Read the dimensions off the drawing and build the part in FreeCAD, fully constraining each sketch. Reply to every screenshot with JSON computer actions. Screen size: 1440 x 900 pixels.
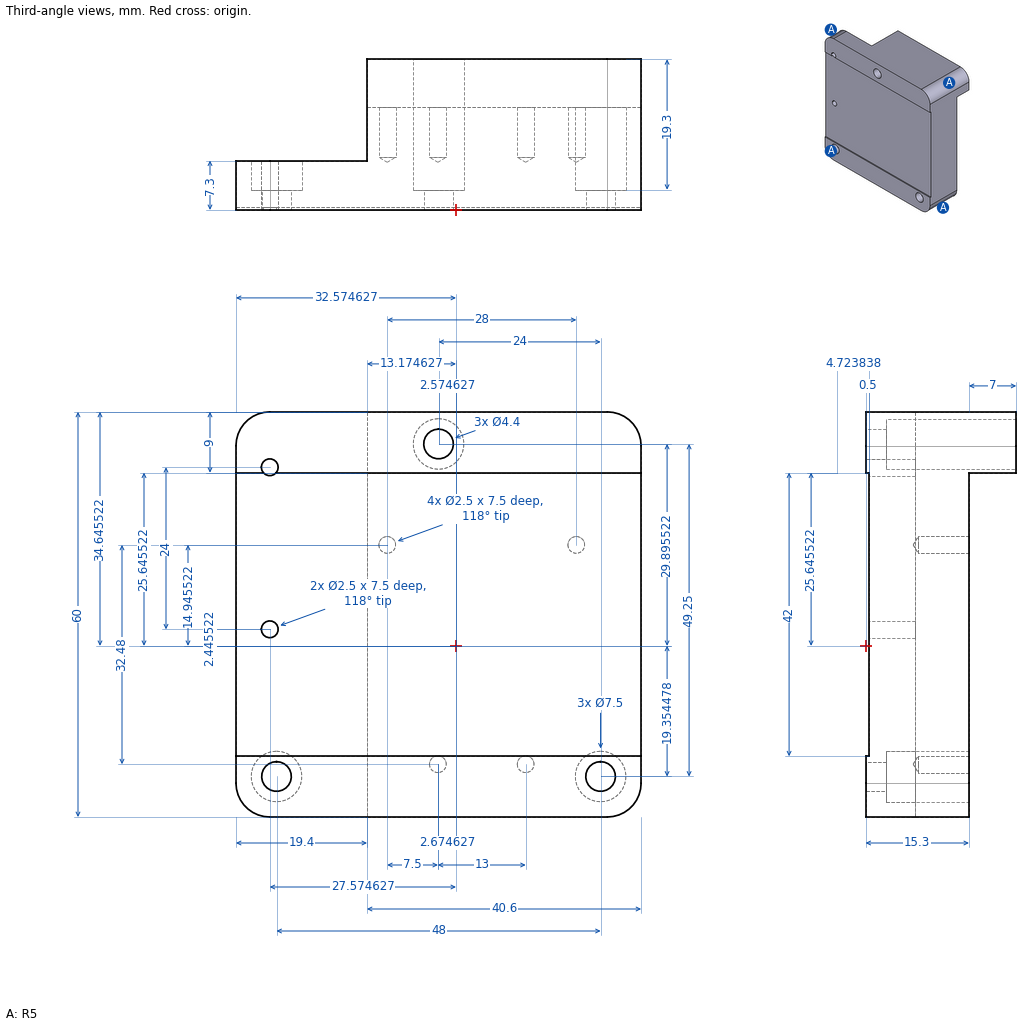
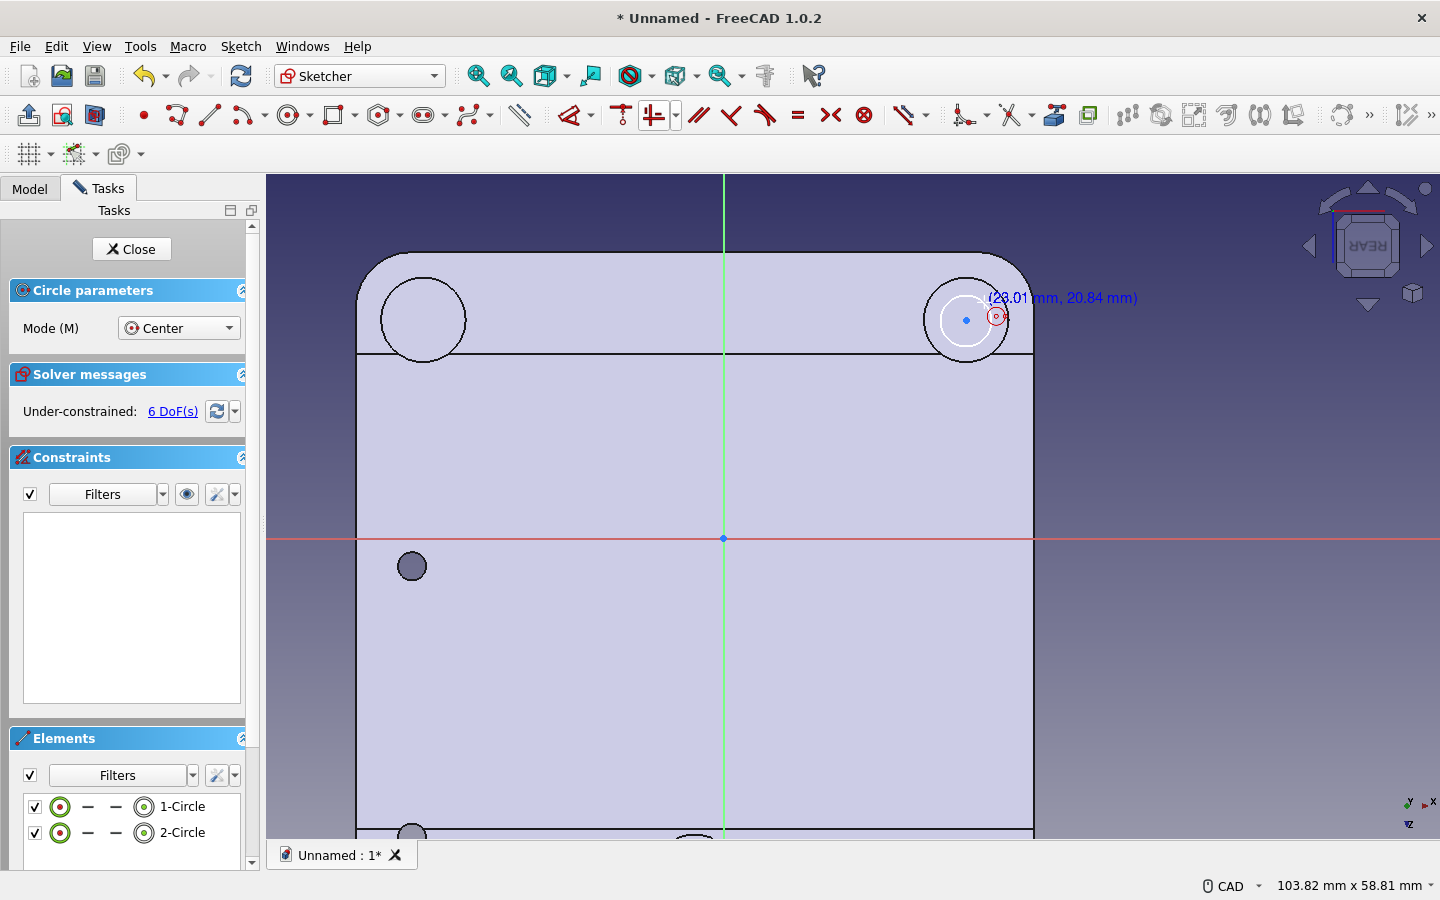
{"action": "left_click", "coordinate": [423, 320]}
{"action": "left_click", "coordinate": [441, 302]}
{"action": "key", "text": "Escape"}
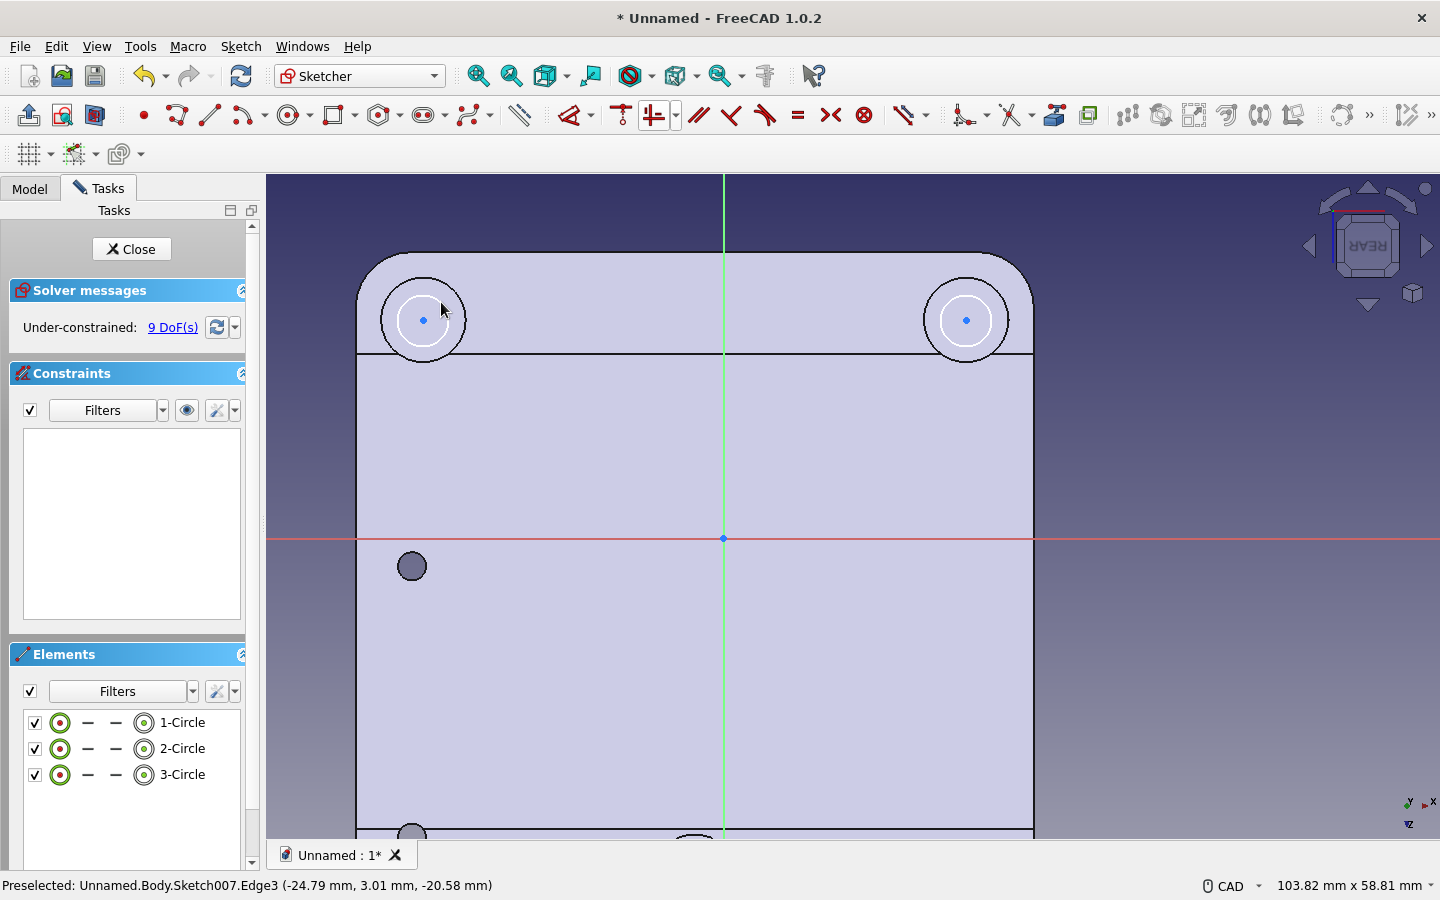
{"action": "scroll", "coordinate": [967, 320], "scroll_direction": "down", "scroll_amount": 2}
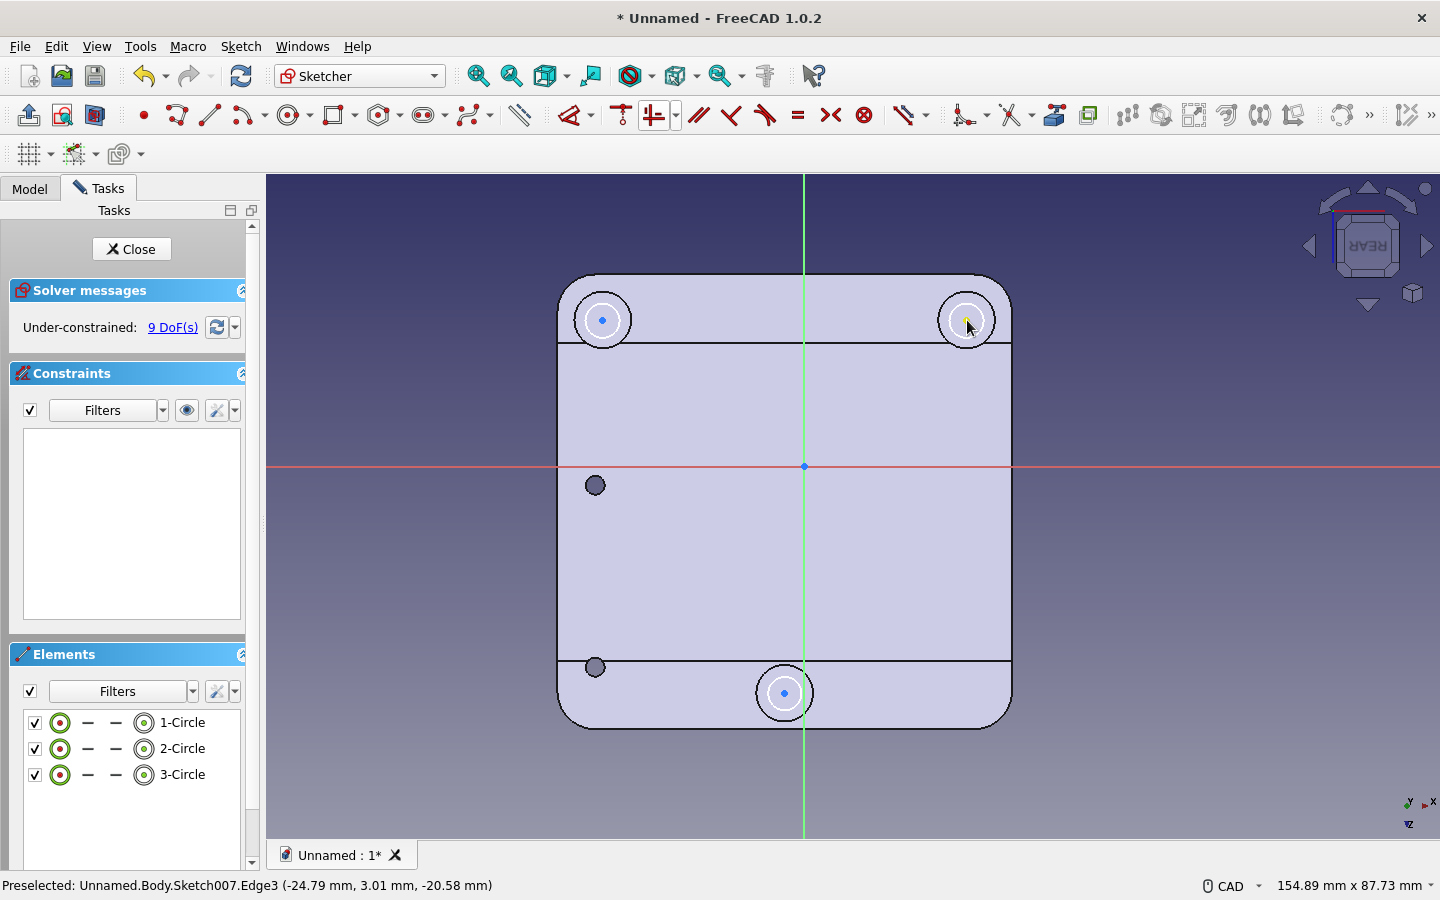
{"action": "scroll", "coordinate": [797, 682], "scroll_direction": "up", "scroll_amount": 3}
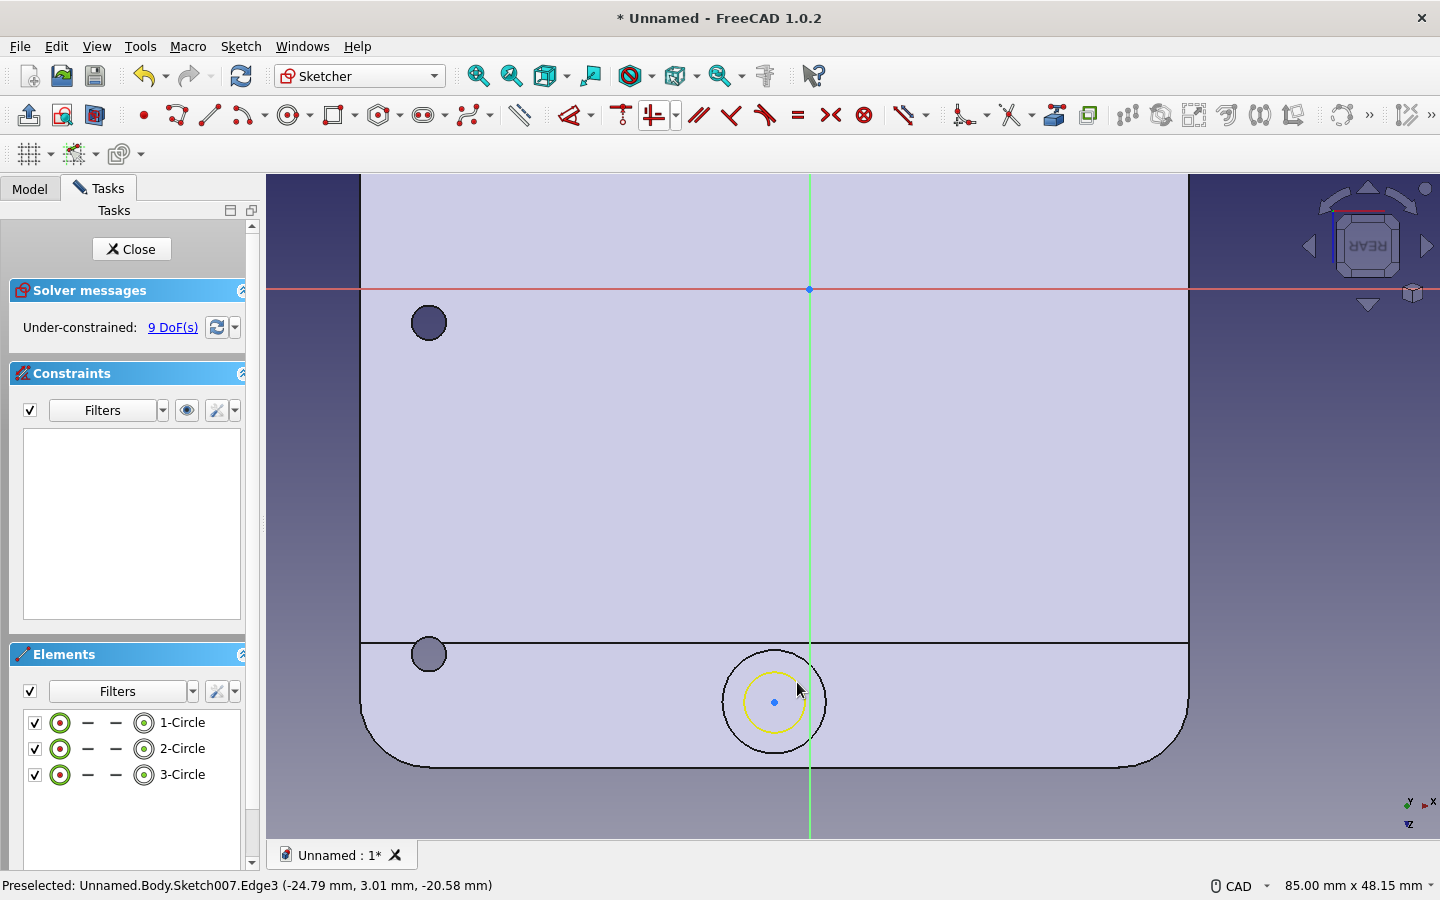
{"action": "left_click", "coordinate": [796, 681]}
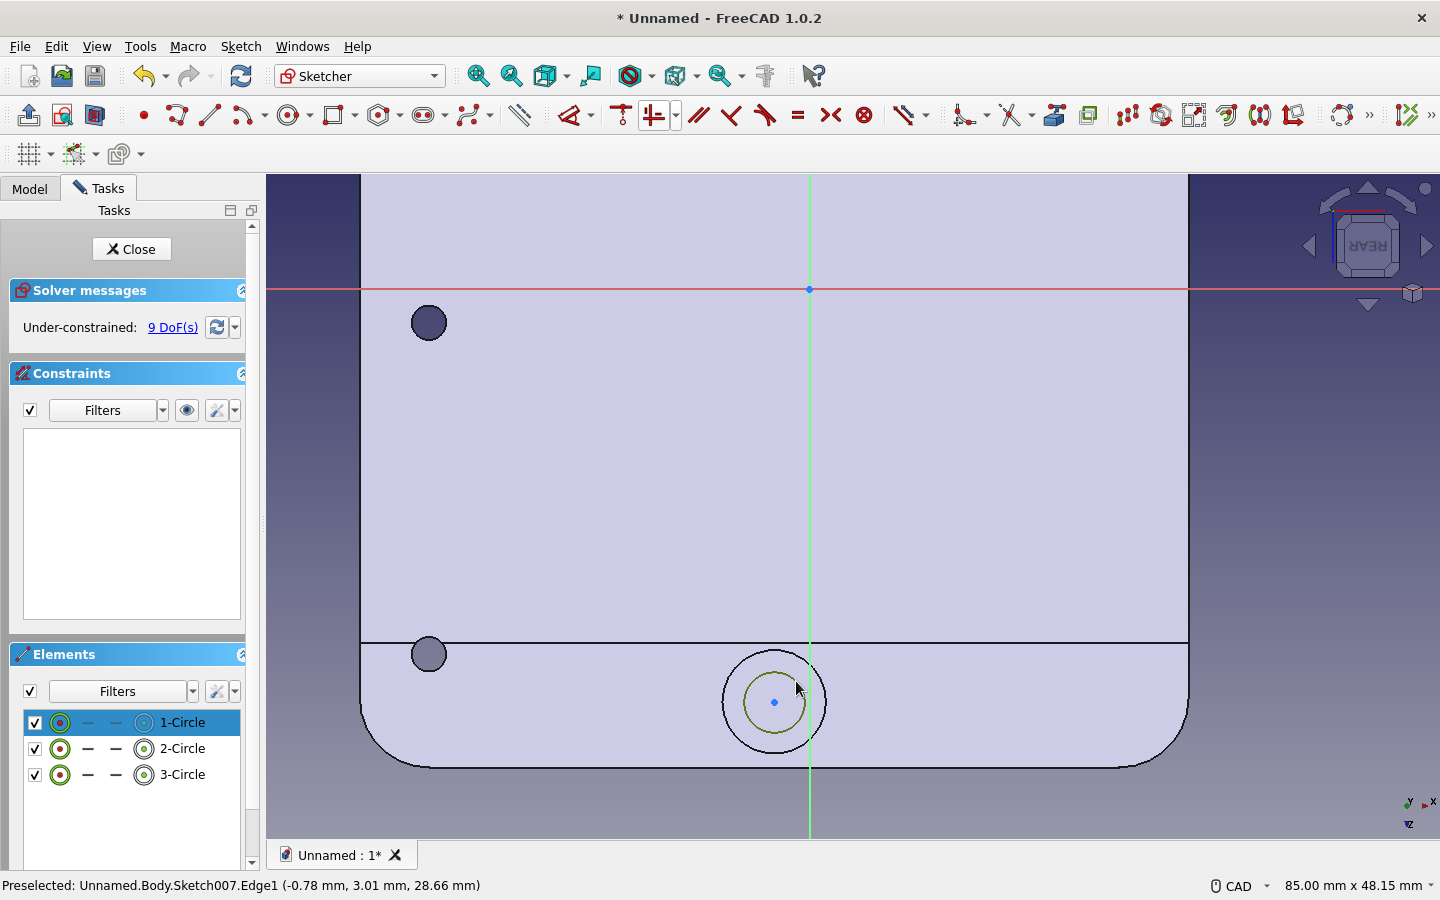
{"action": "scroll", "coordinate": [797, 683], "scroll_direction": "down", "scroll_amount": 3}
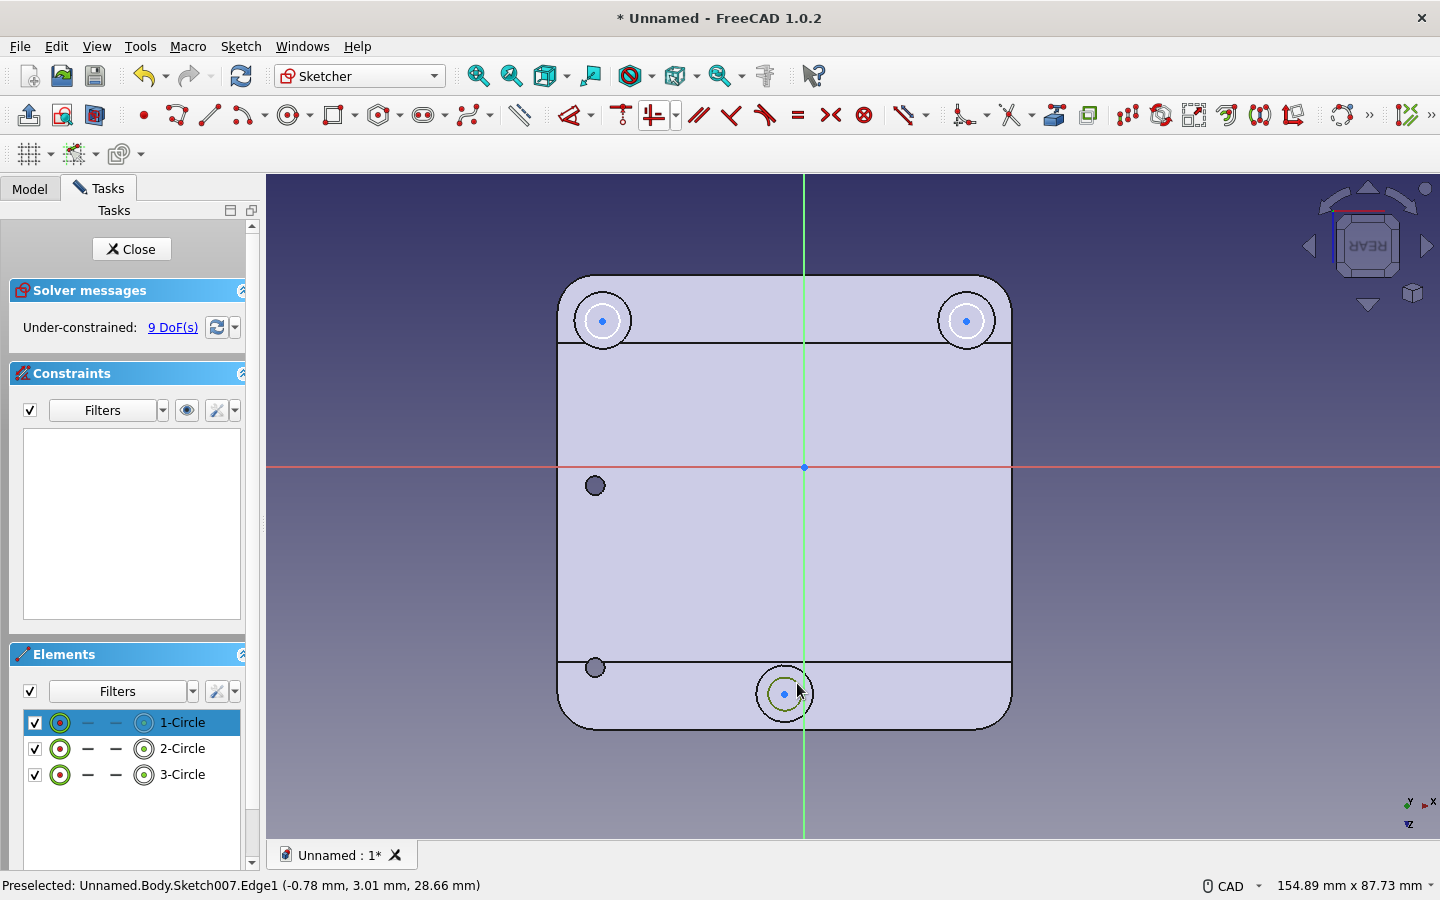
{"action": "left_click", "coordinate": [979, 309]}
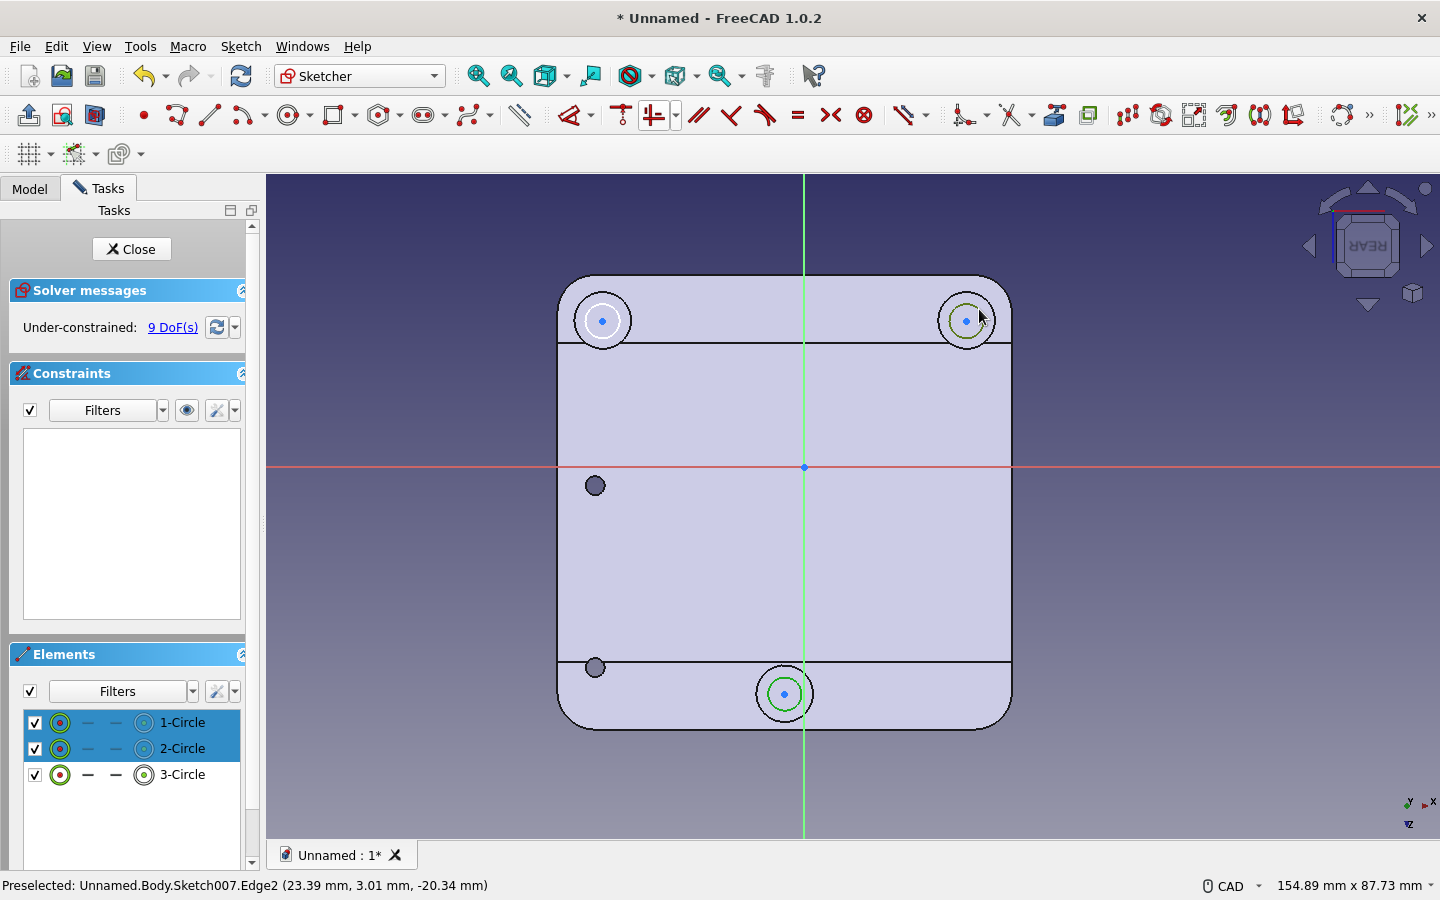
{"action": "left_click", "coordinate": [615, 309]}